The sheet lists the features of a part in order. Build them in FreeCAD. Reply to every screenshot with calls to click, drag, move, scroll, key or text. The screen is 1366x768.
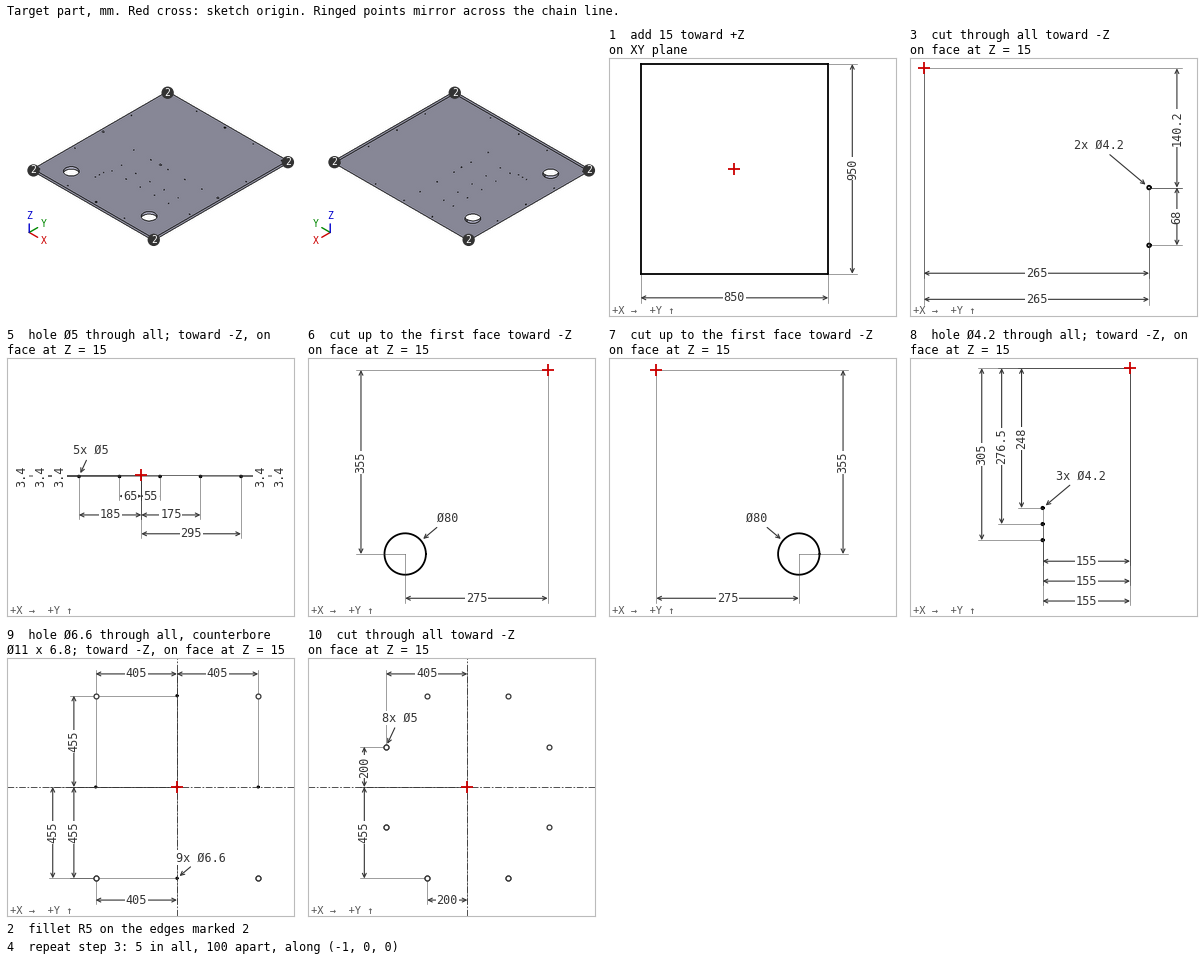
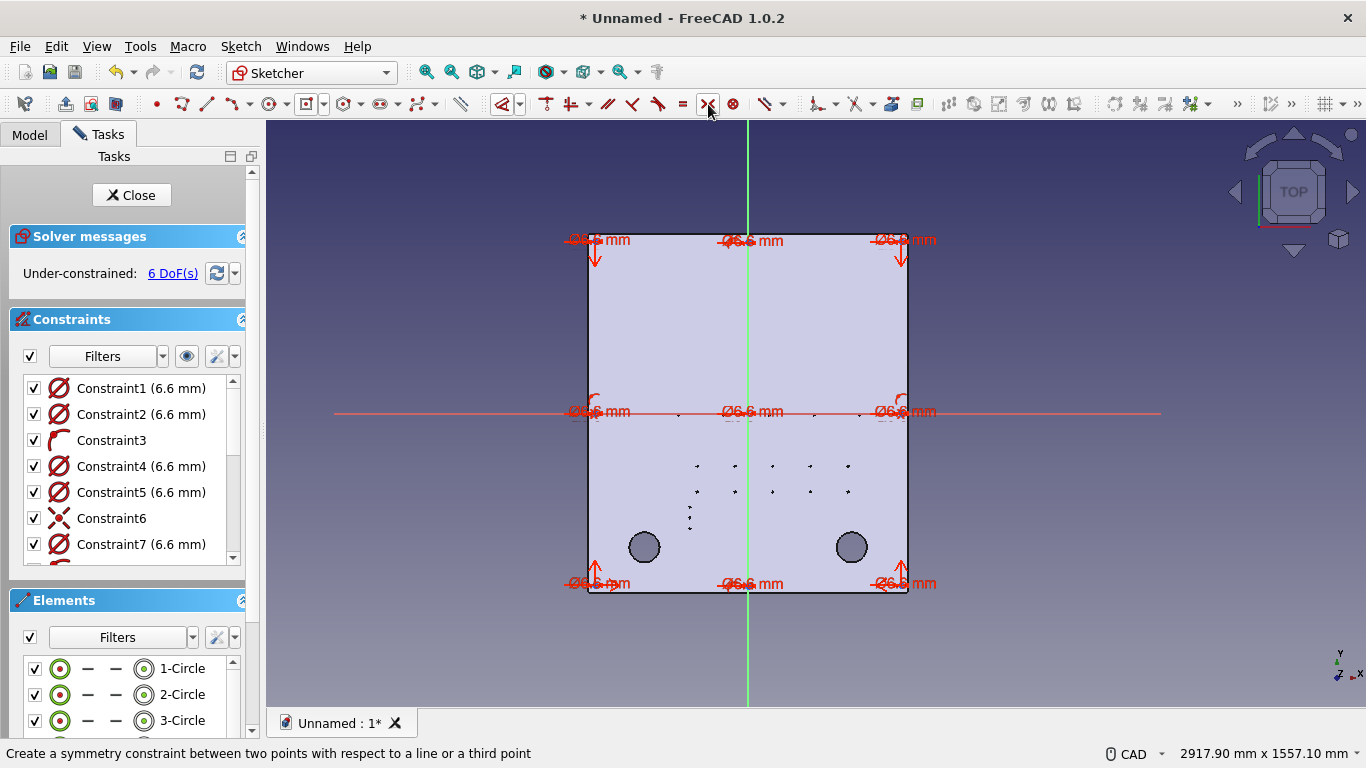
click(595, 585)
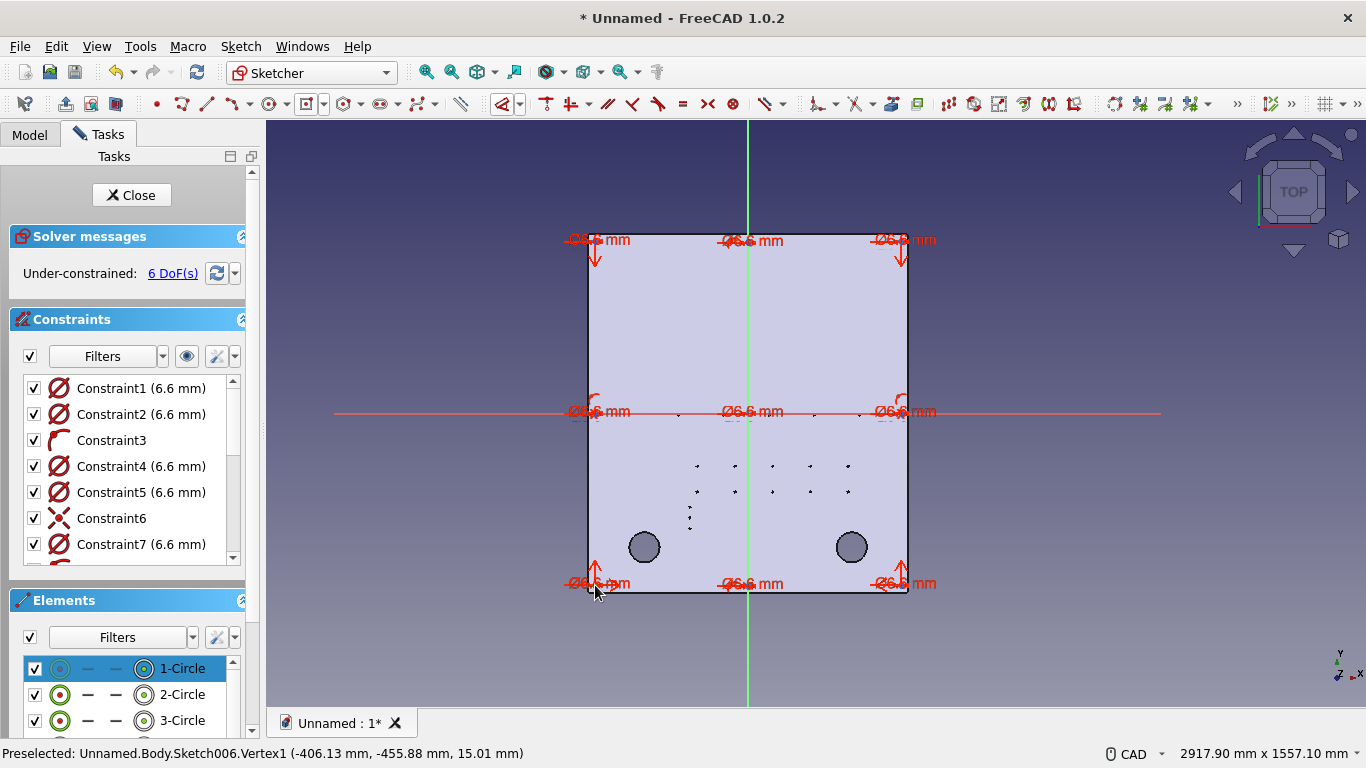
click(520, 104)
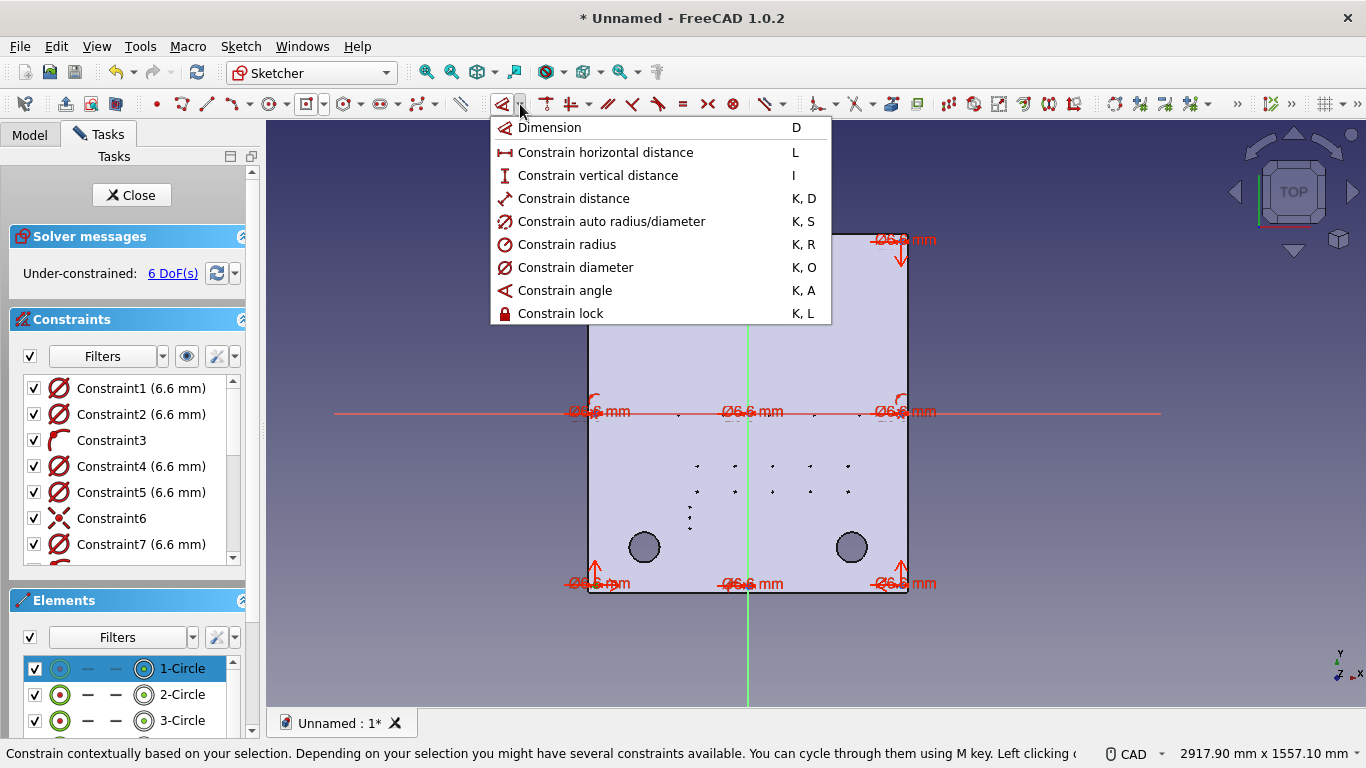
click(661, 152)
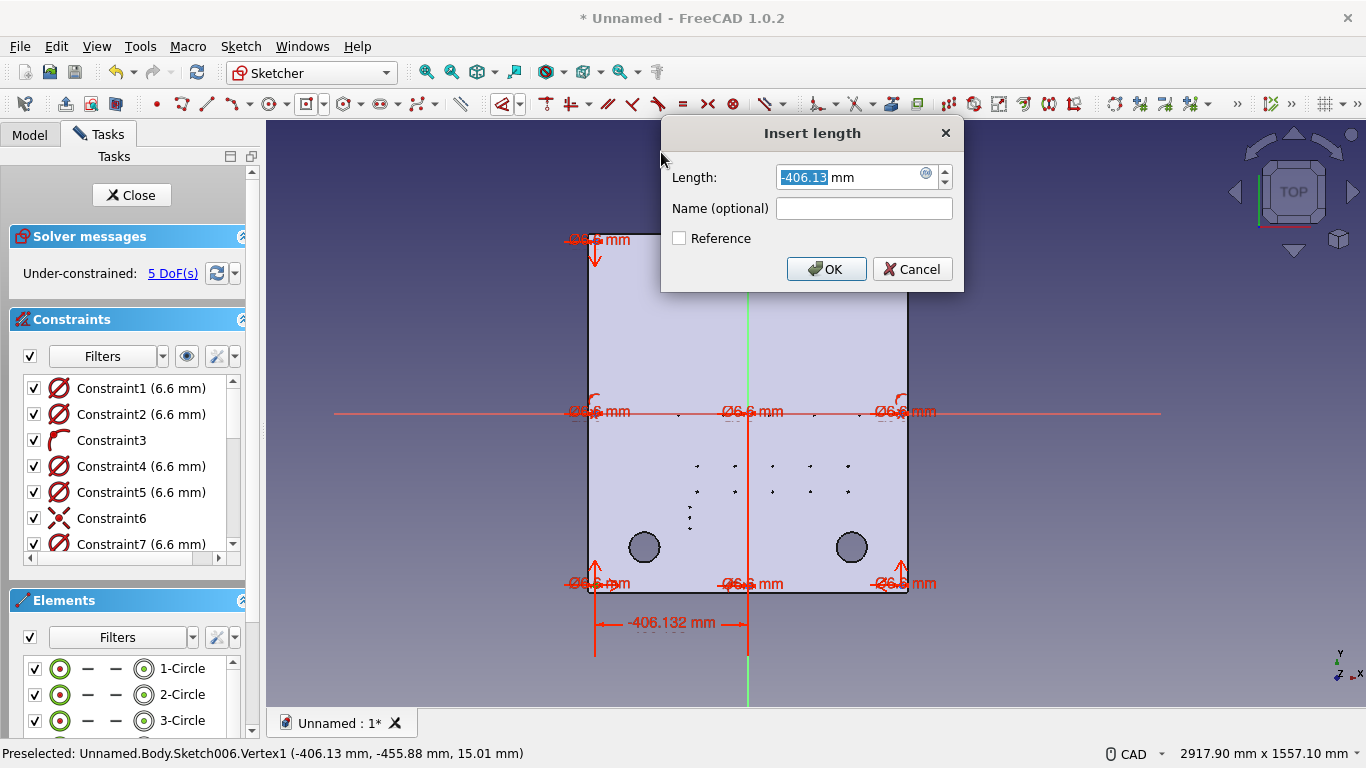
text(-405)
key(Return)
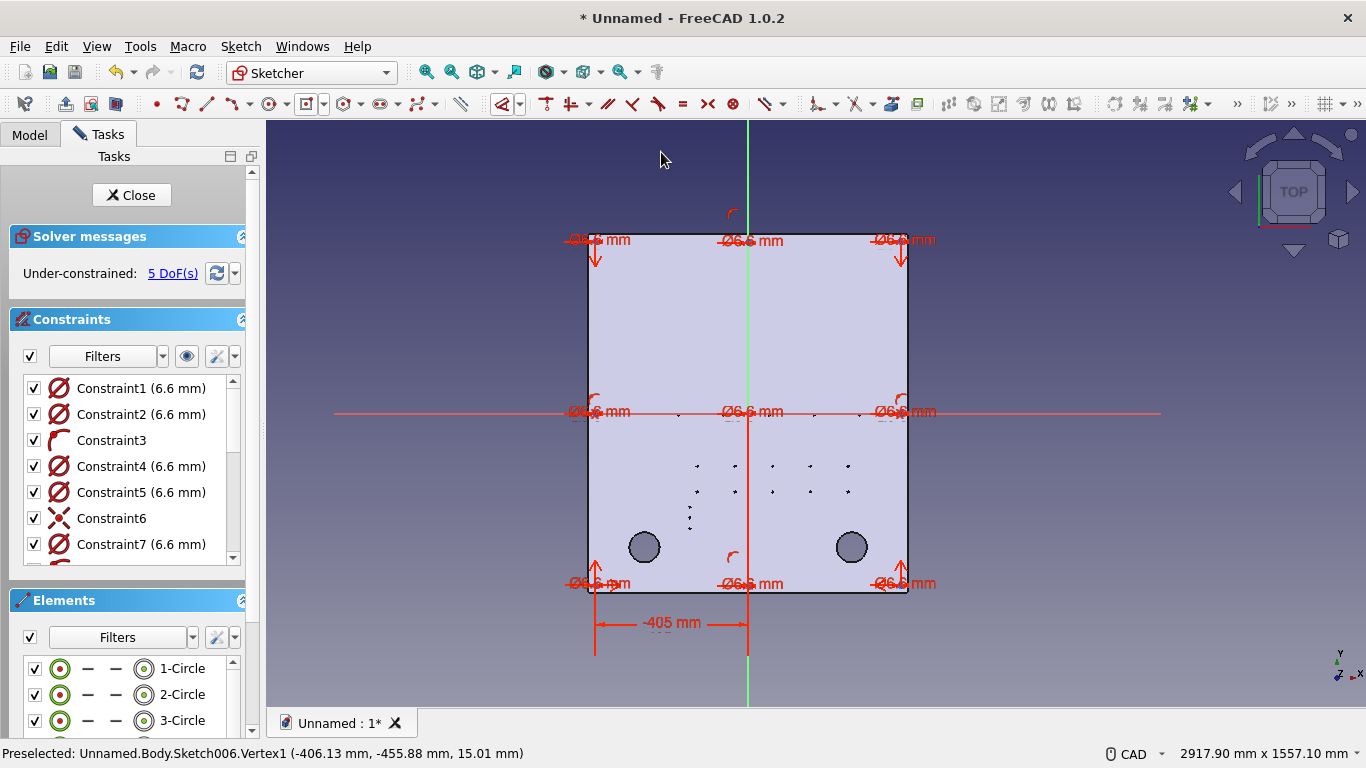
click(595, 585)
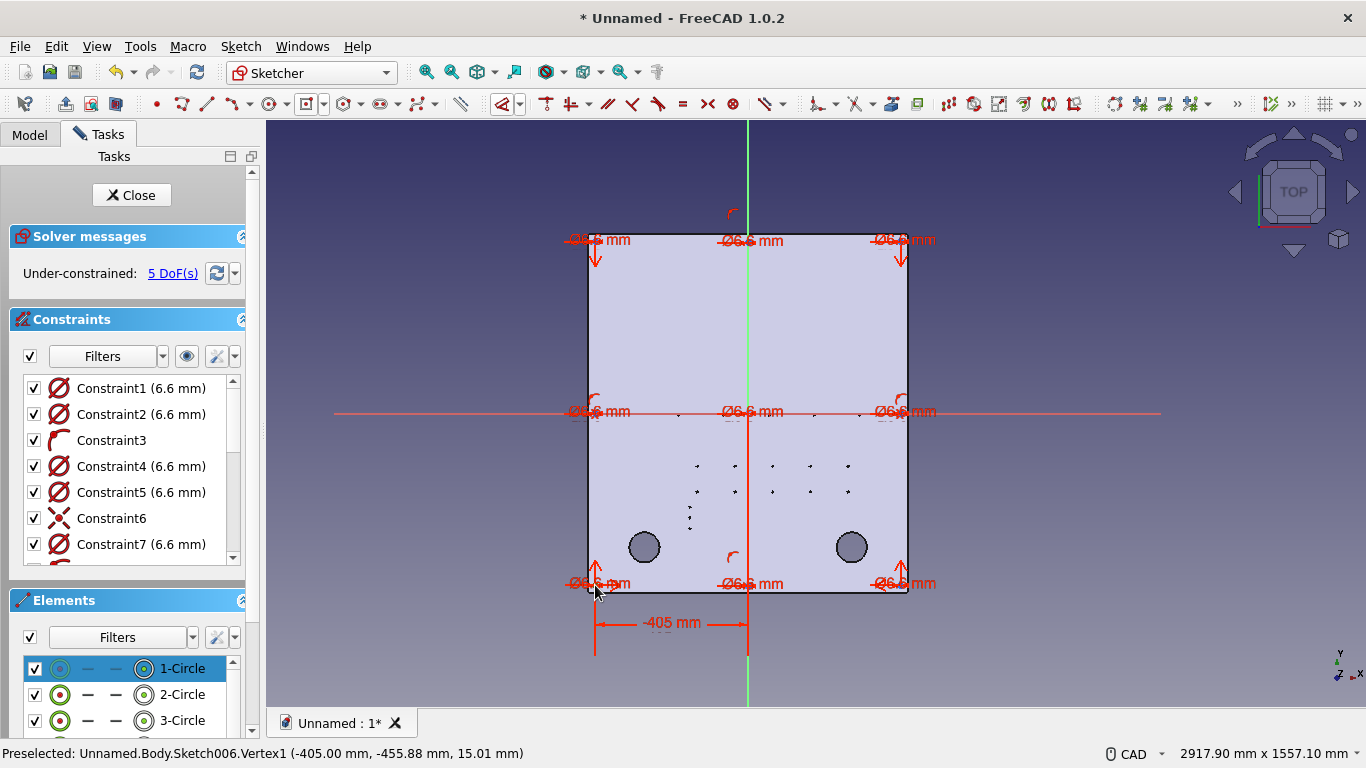
key(i)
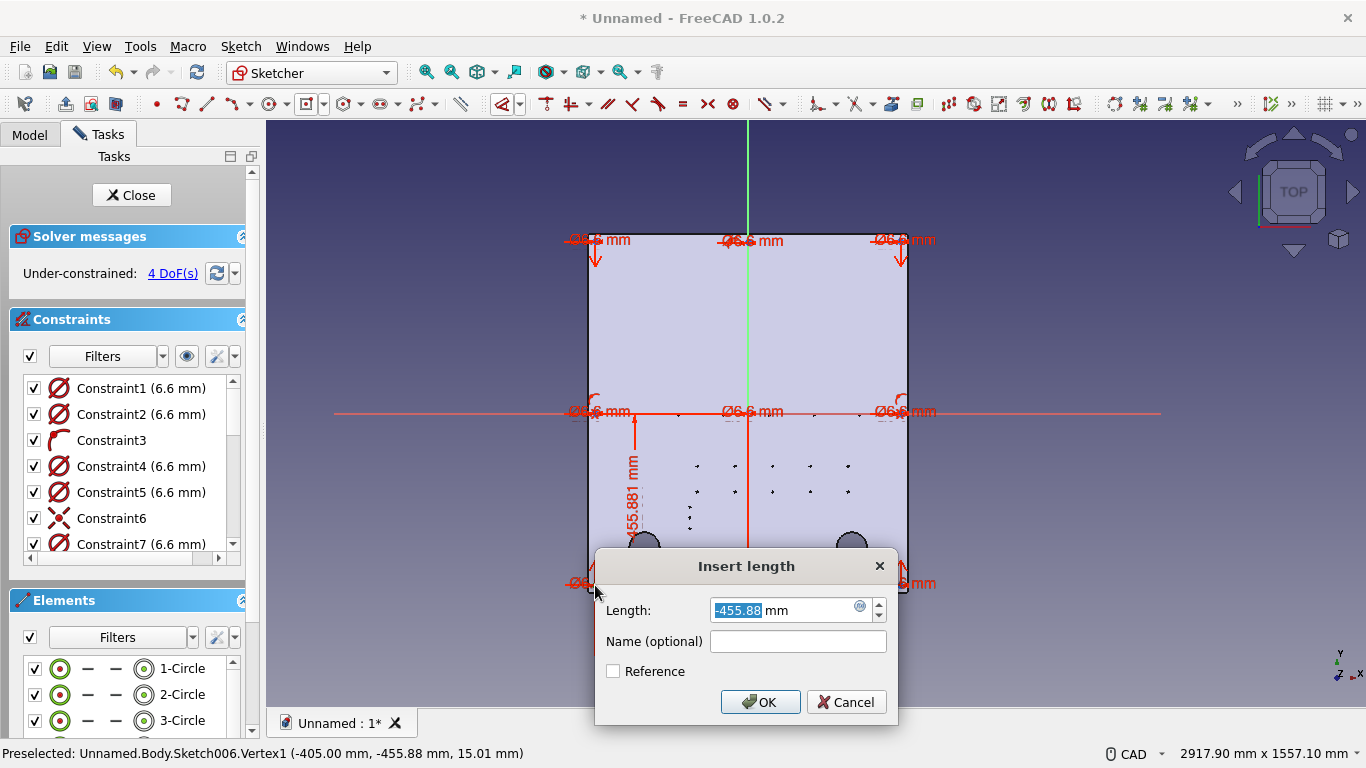
text(-455)
key(Return)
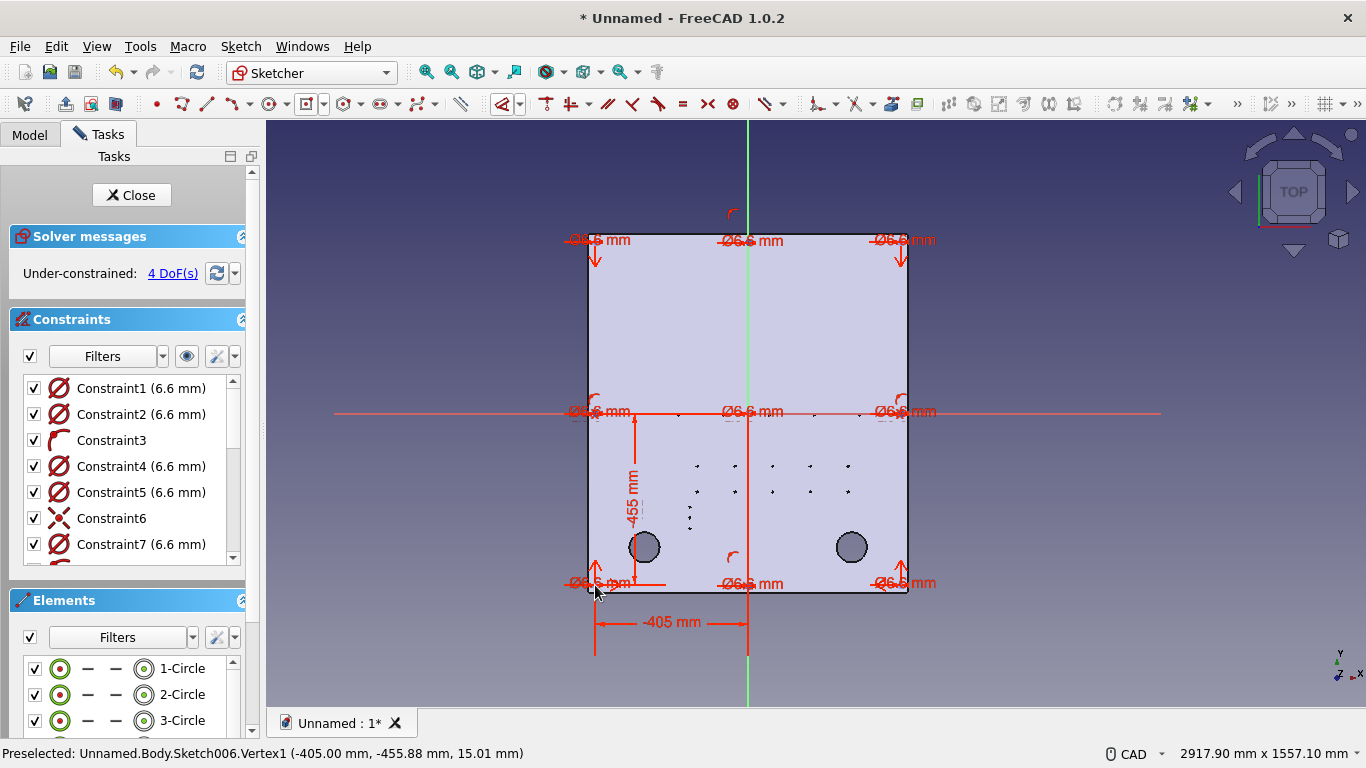
click(748, 586)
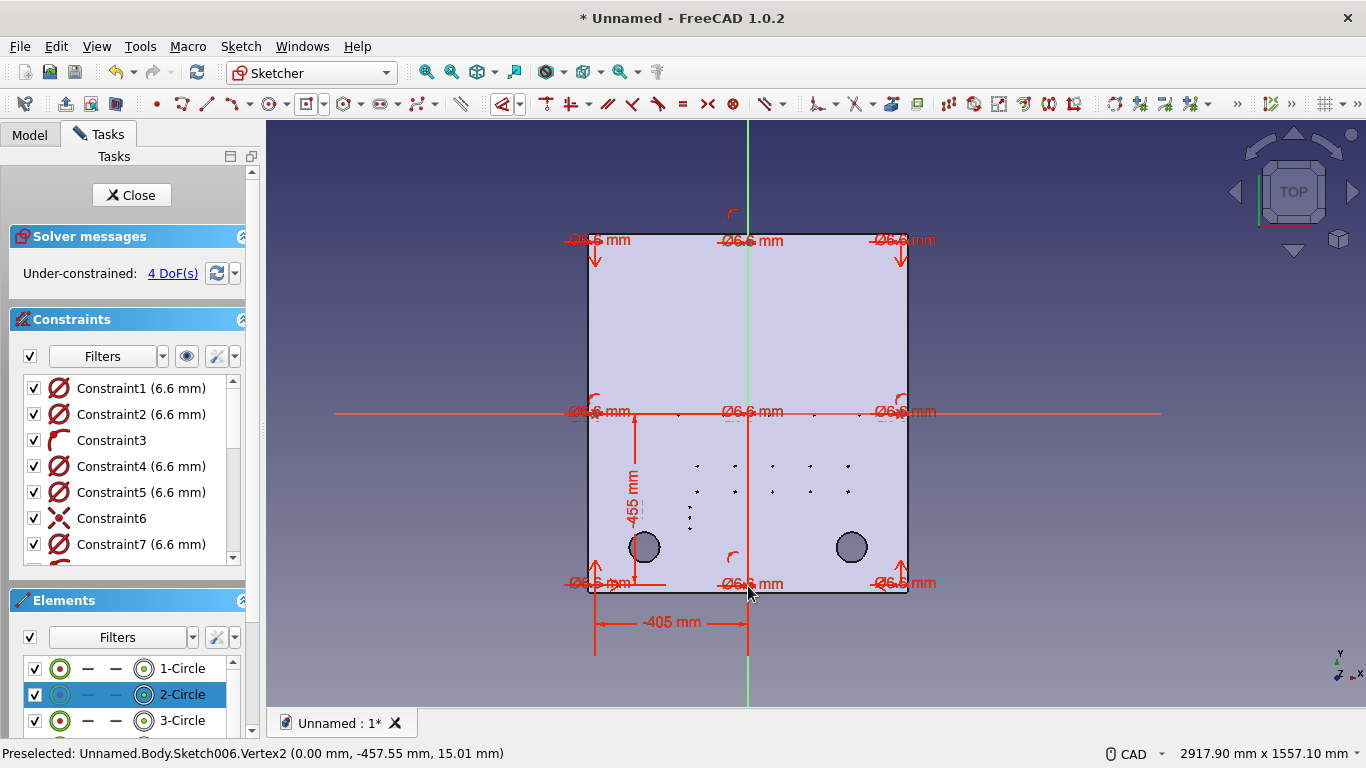
click(520, 104)